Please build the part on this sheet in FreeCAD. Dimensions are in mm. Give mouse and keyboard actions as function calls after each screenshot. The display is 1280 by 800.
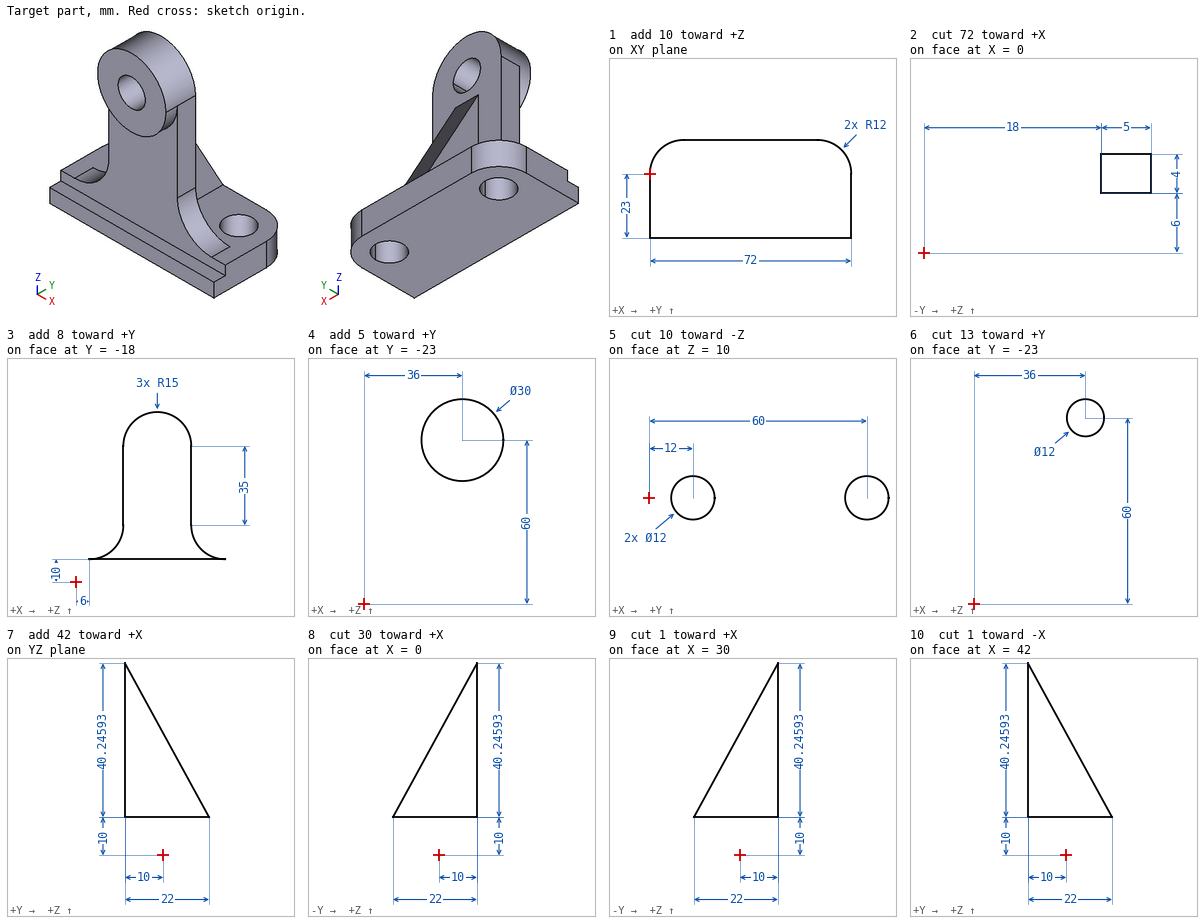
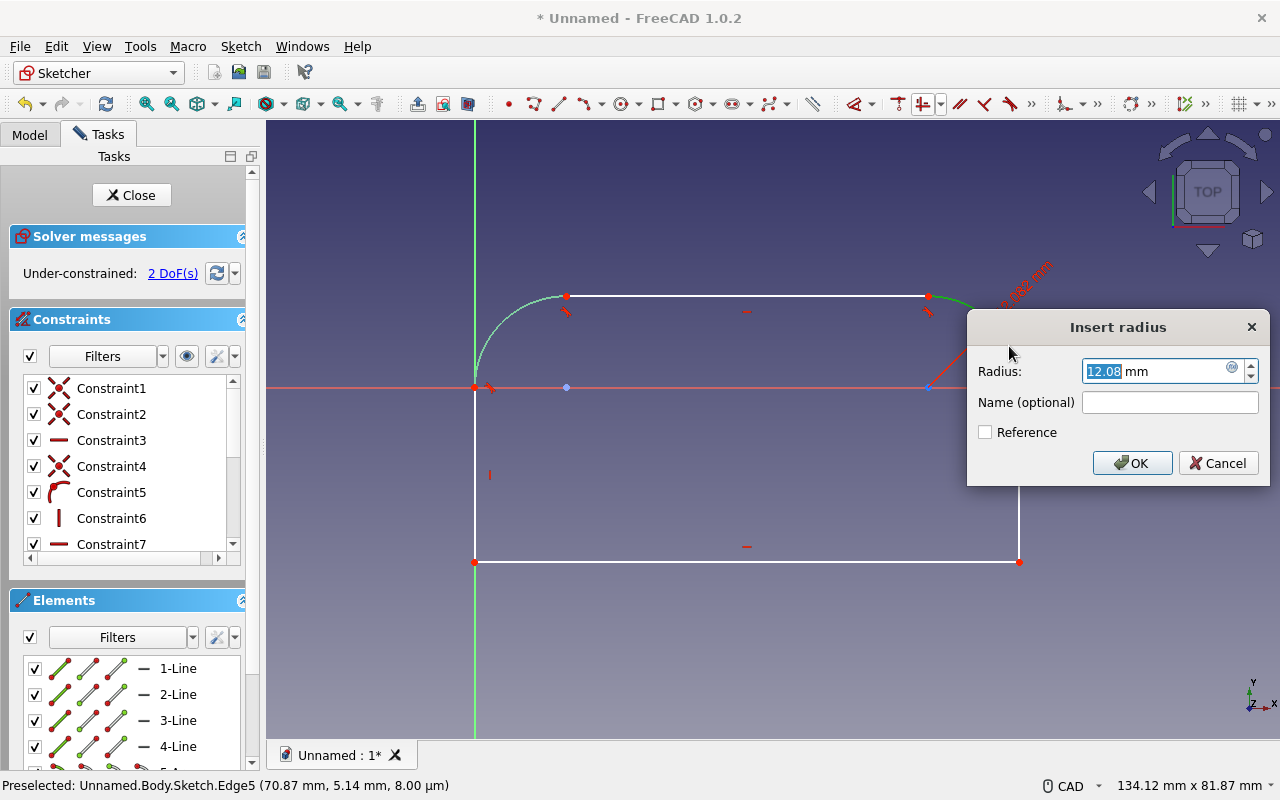
text(12)
key(Return)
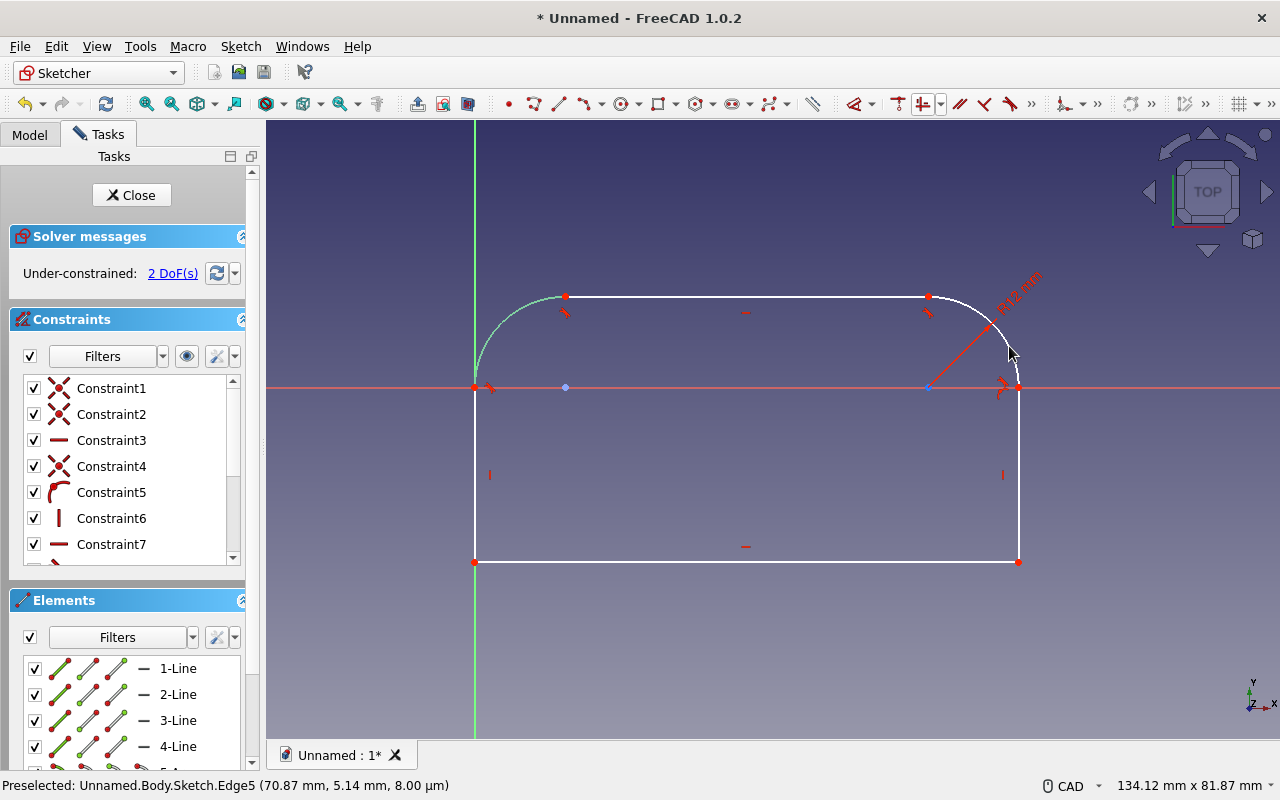
click(475, 440)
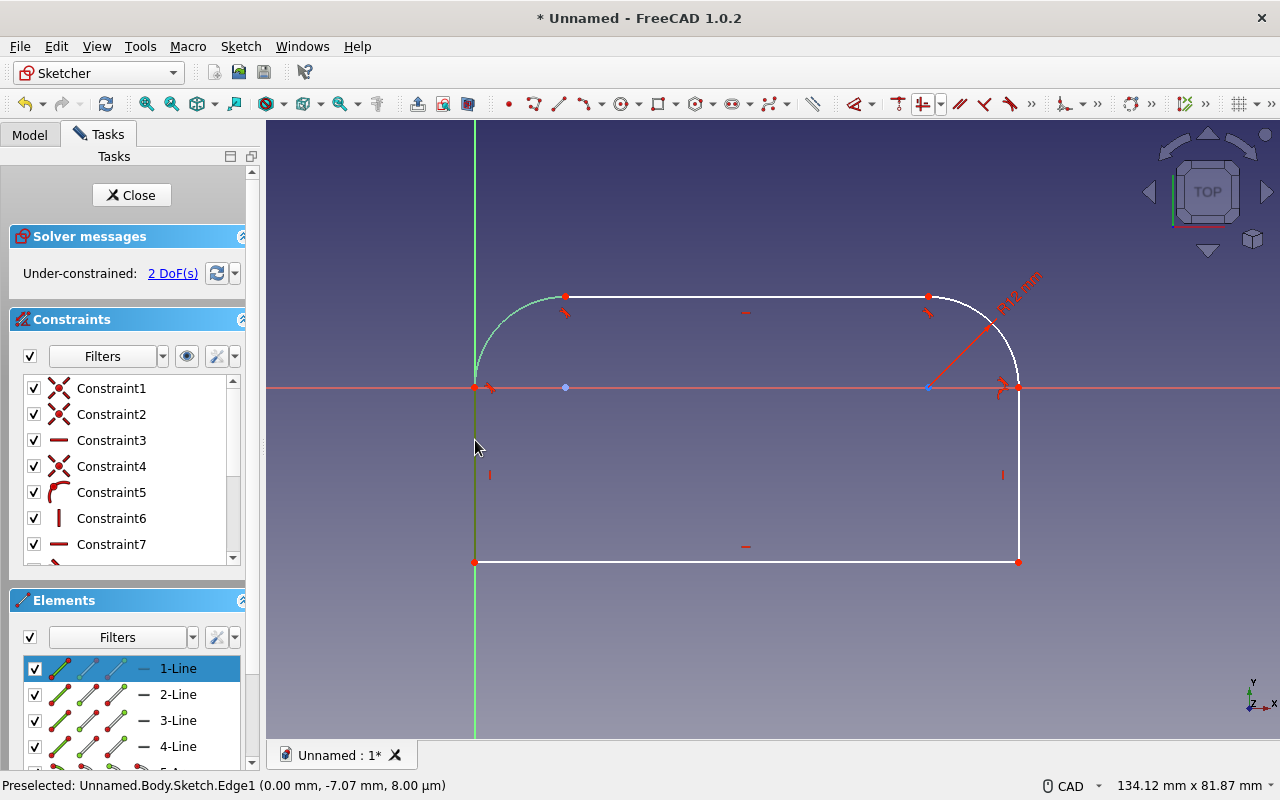
click(872, 104)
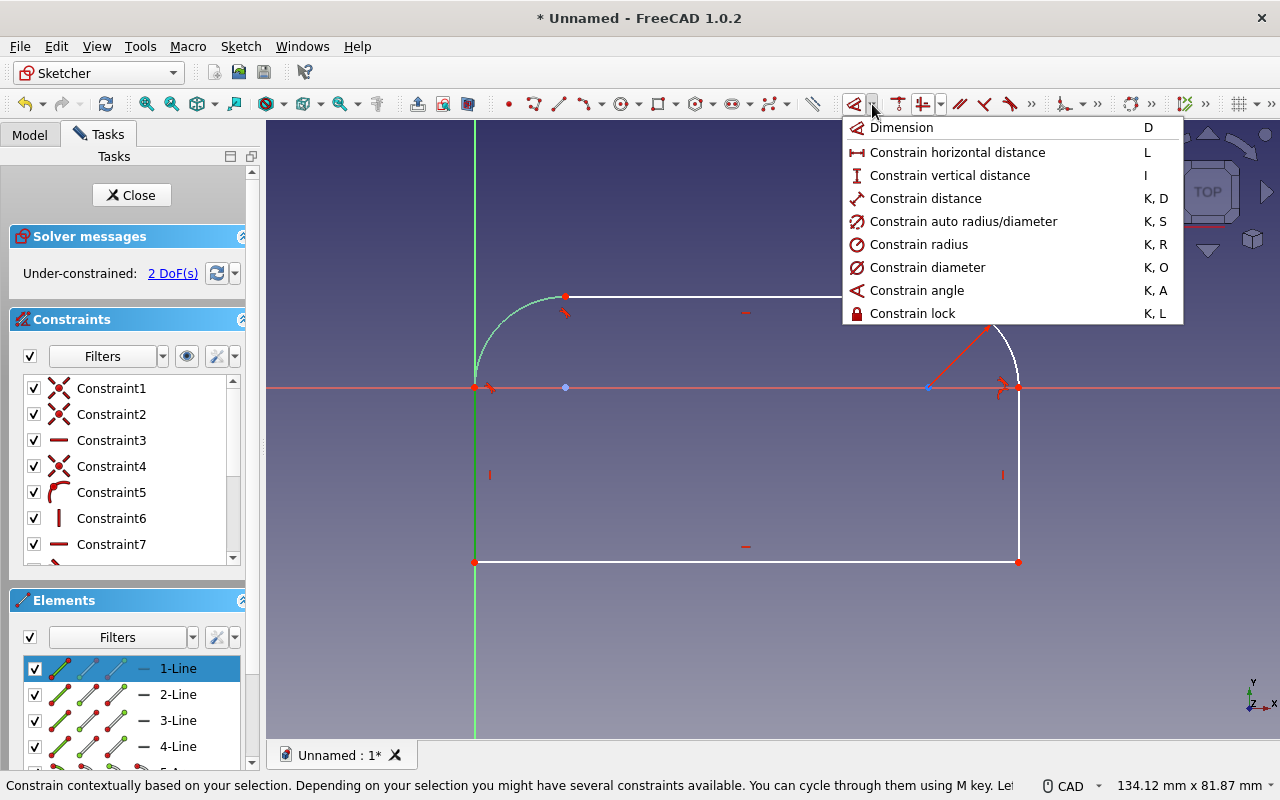
click(1013, 176)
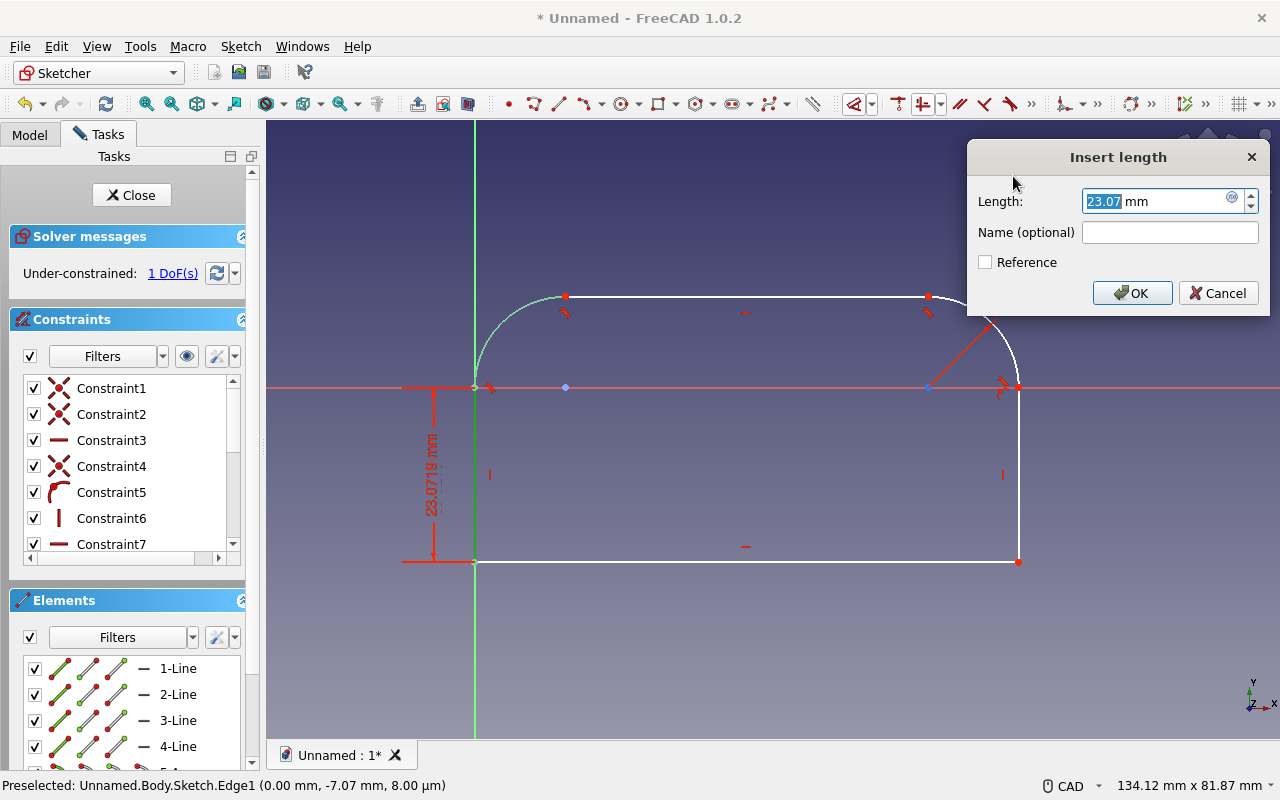
text(23)
key(Return)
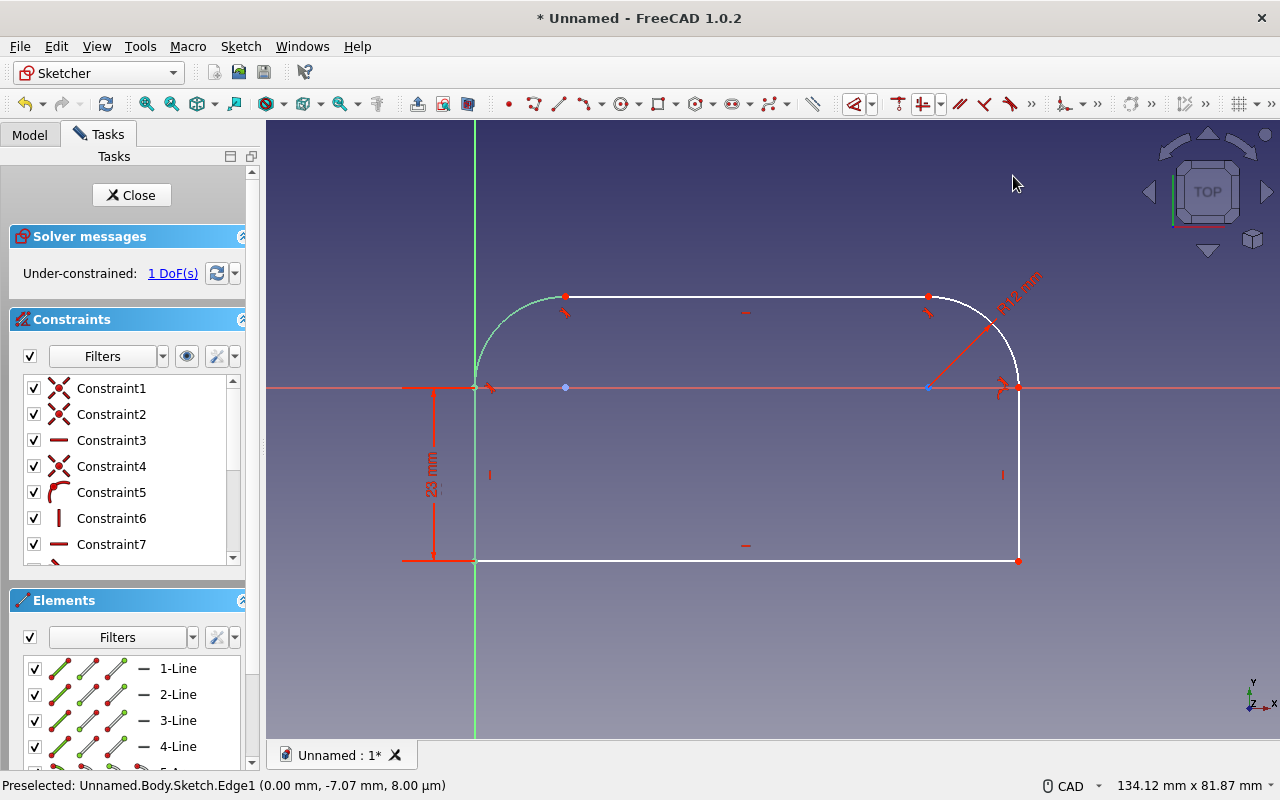
click(638, 561)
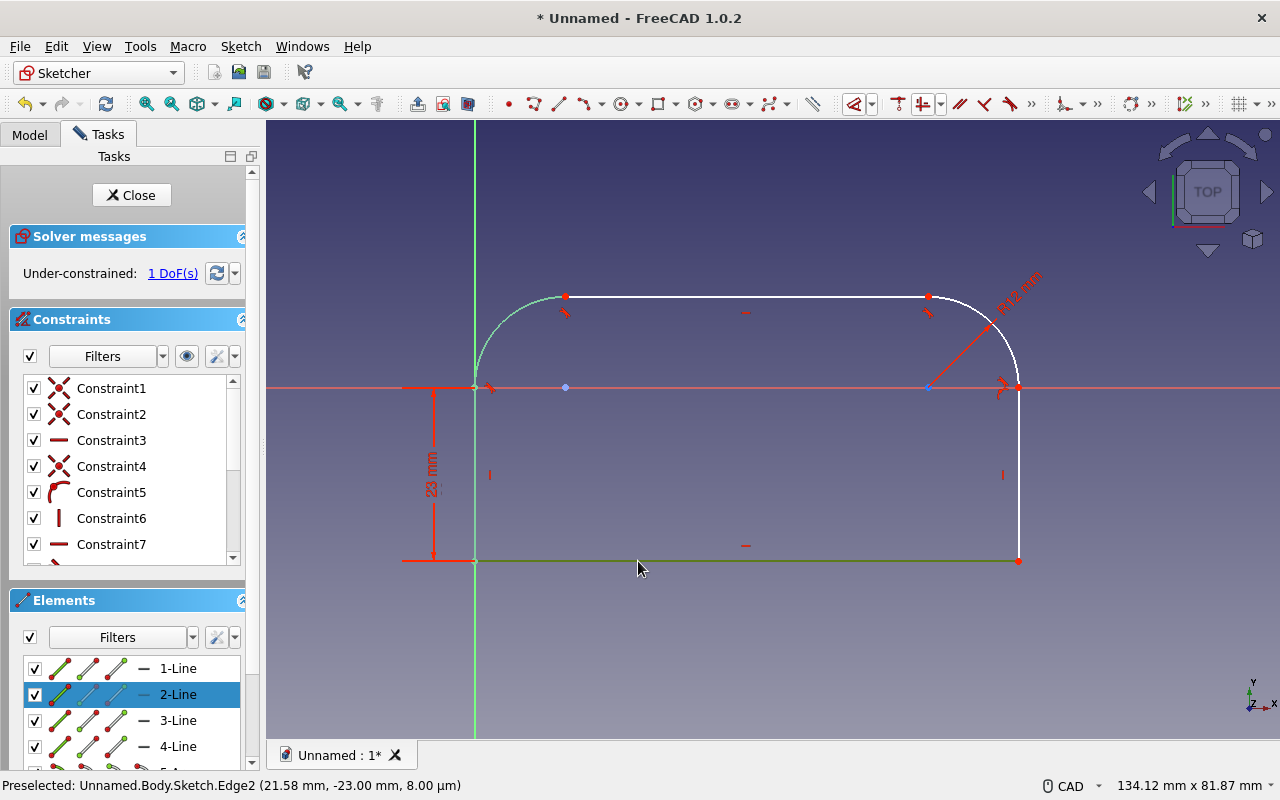
key(l)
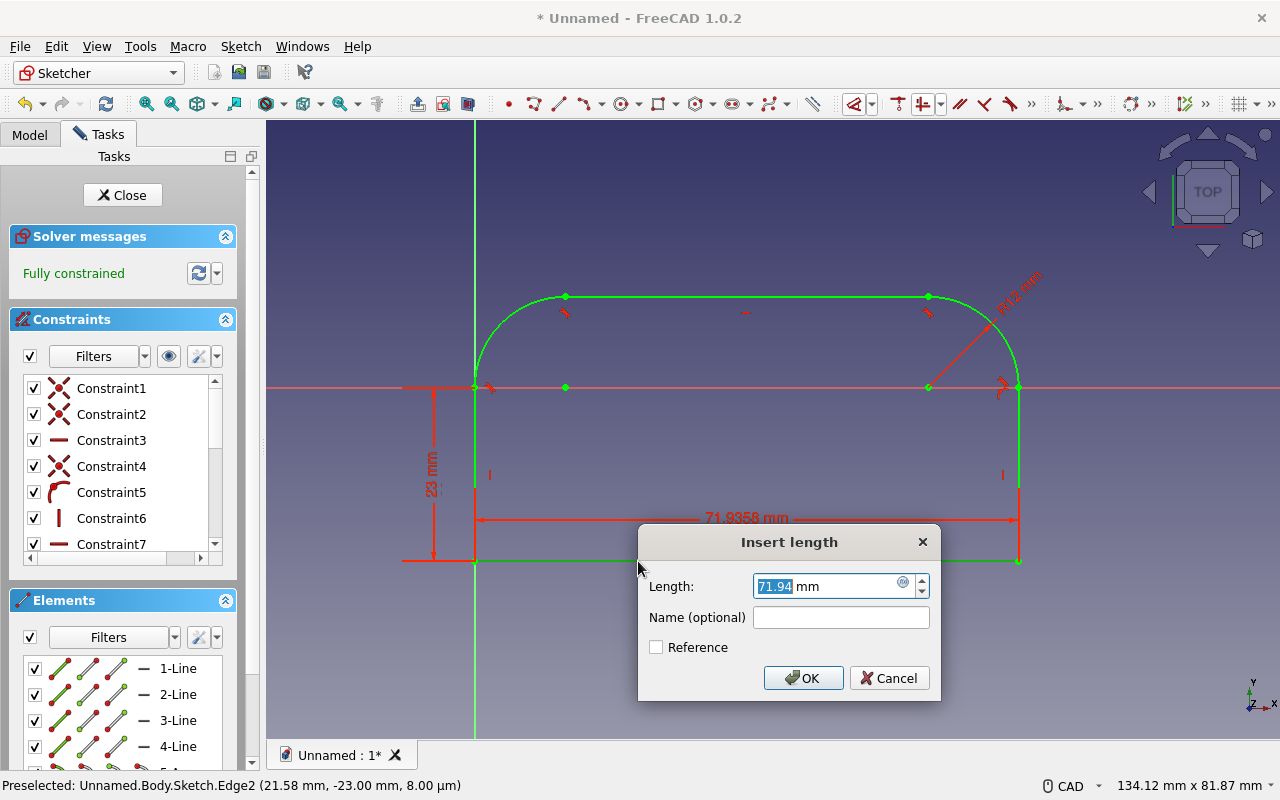
text(72)
key(Return)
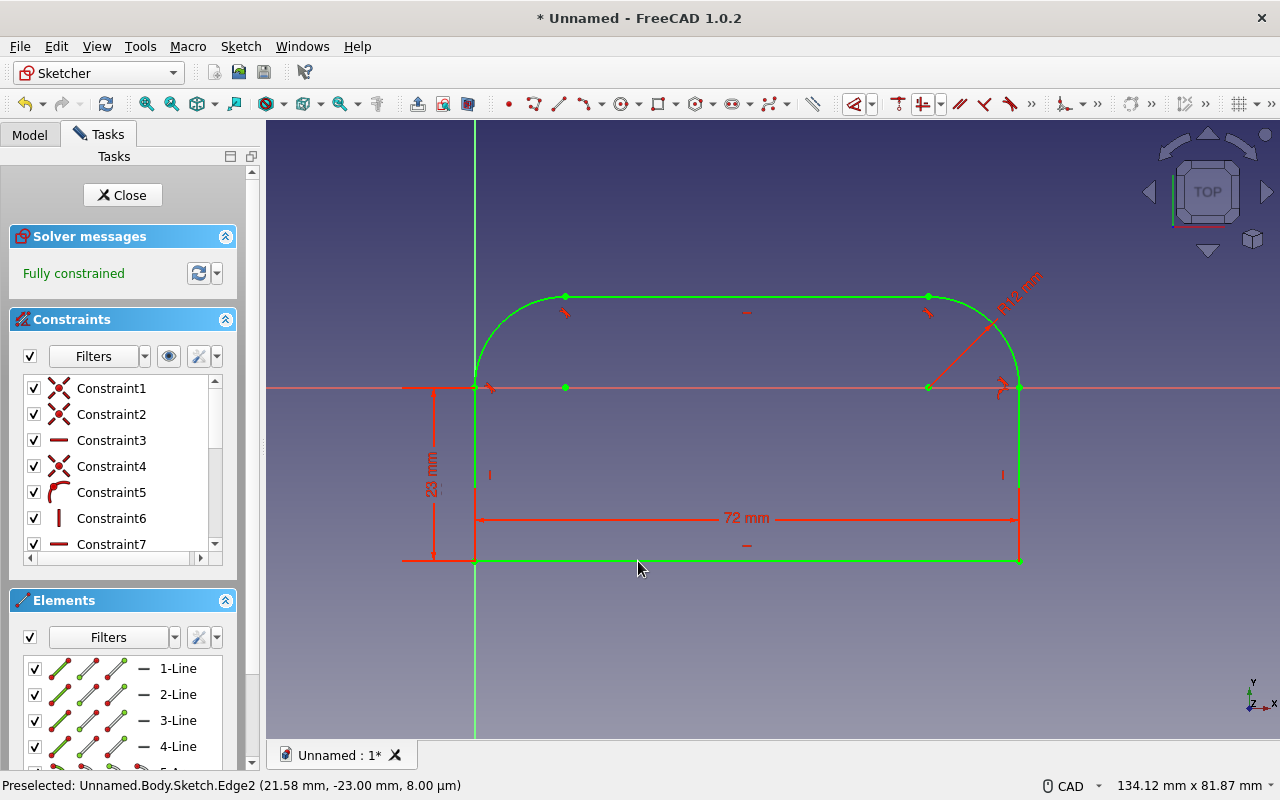
click(123, 195)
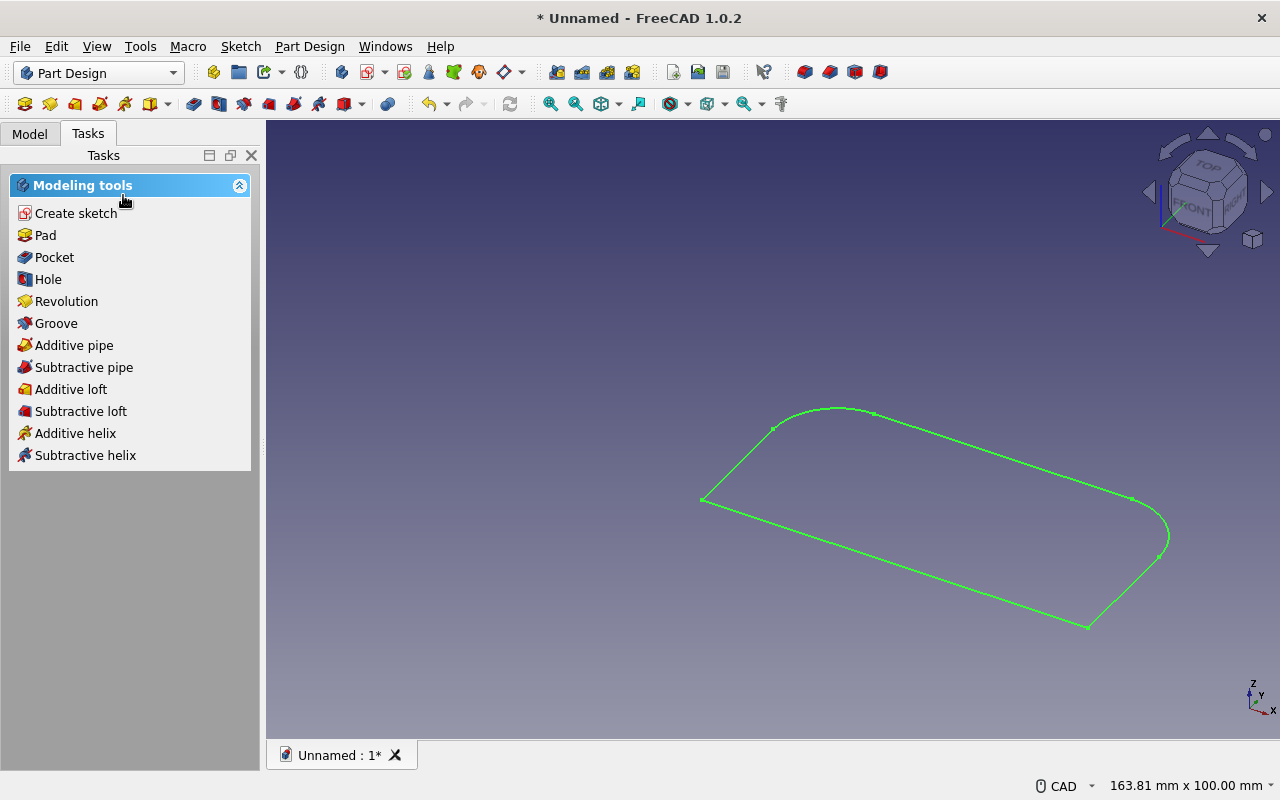
click(25, 104)